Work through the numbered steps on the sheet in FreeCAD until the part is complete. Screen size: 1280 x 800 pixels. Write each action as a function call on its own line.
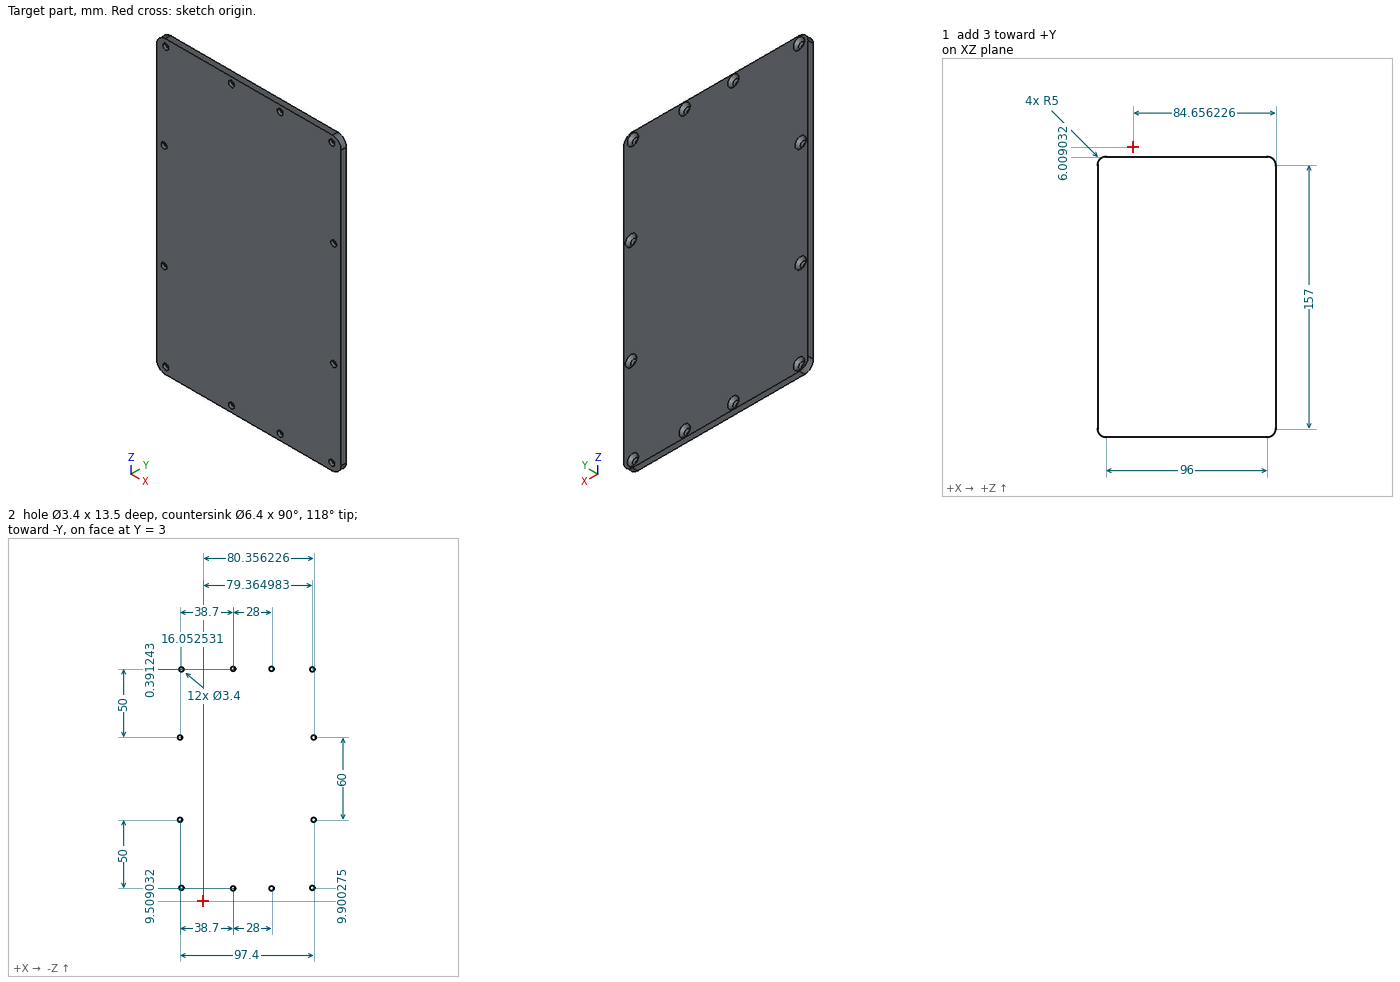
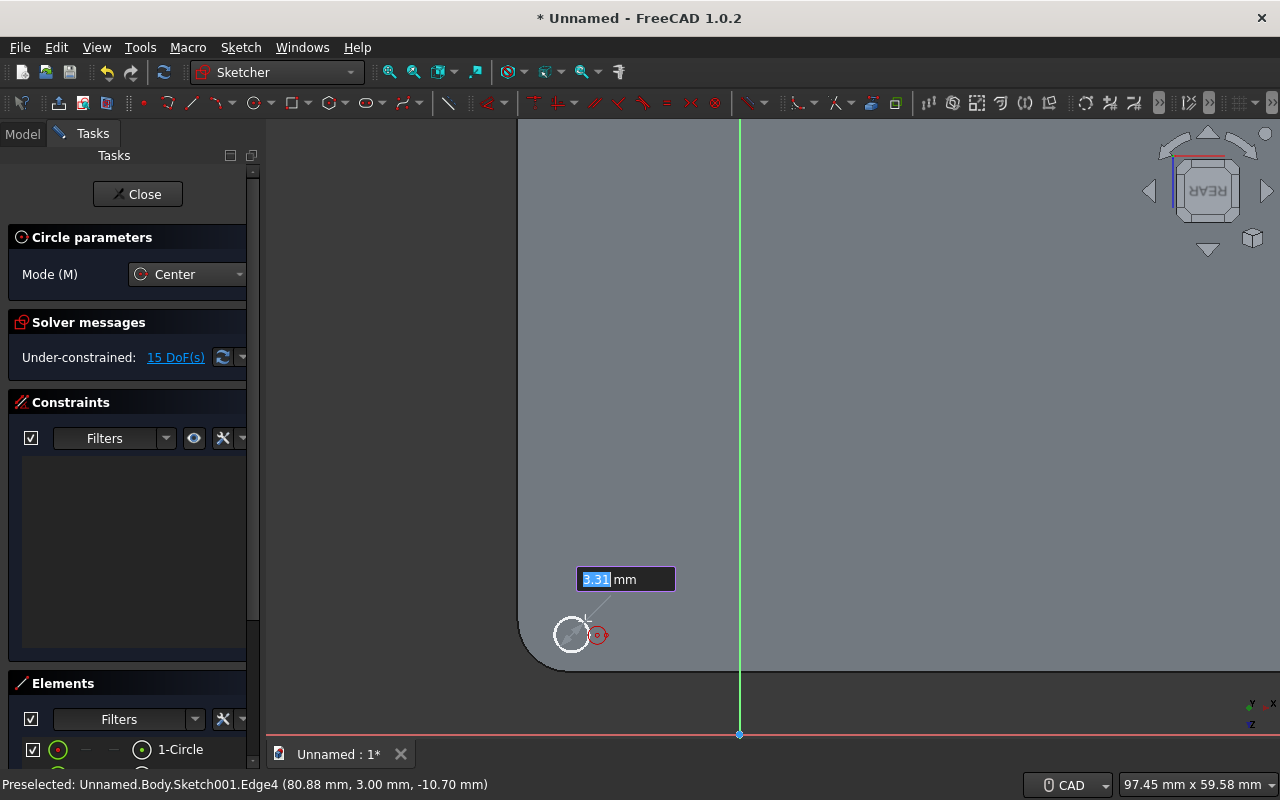
click(585, 619)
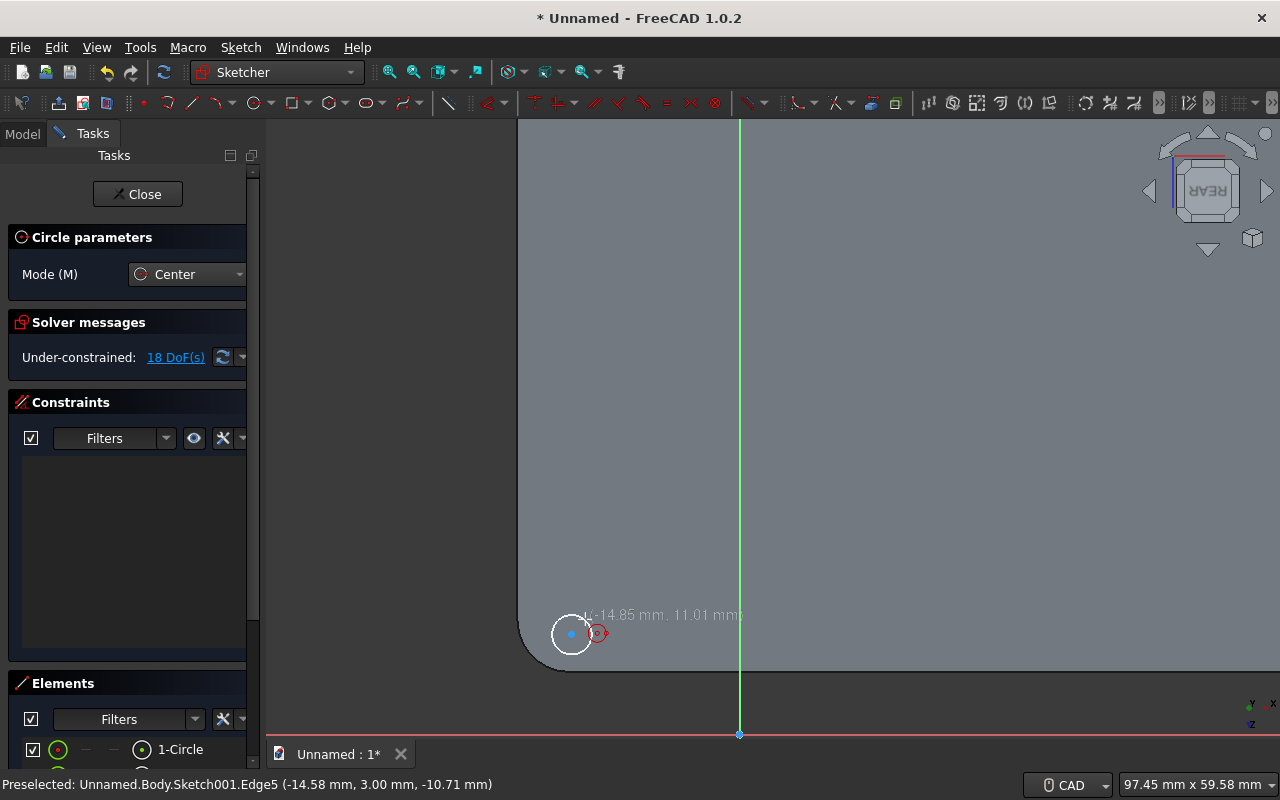
scroll(585, 621, down, 7)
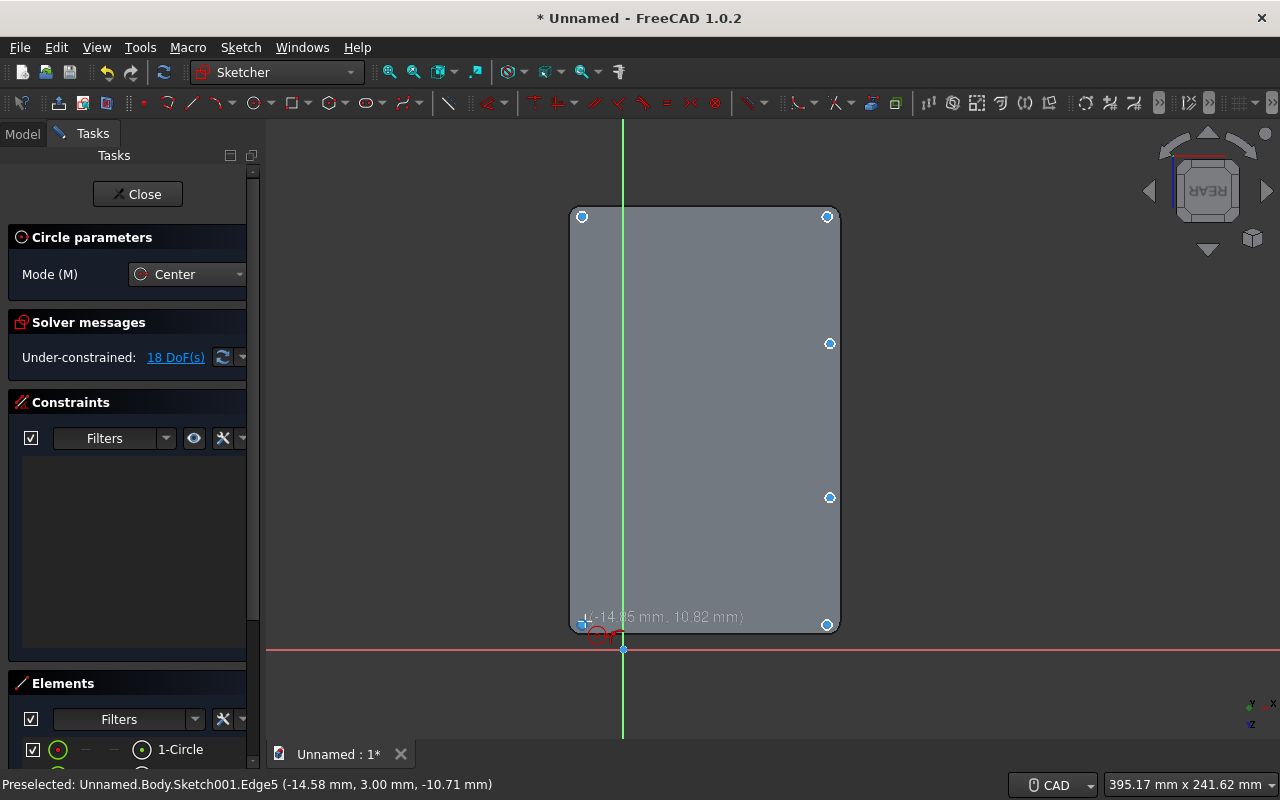
scroll(580, 497, up, 9)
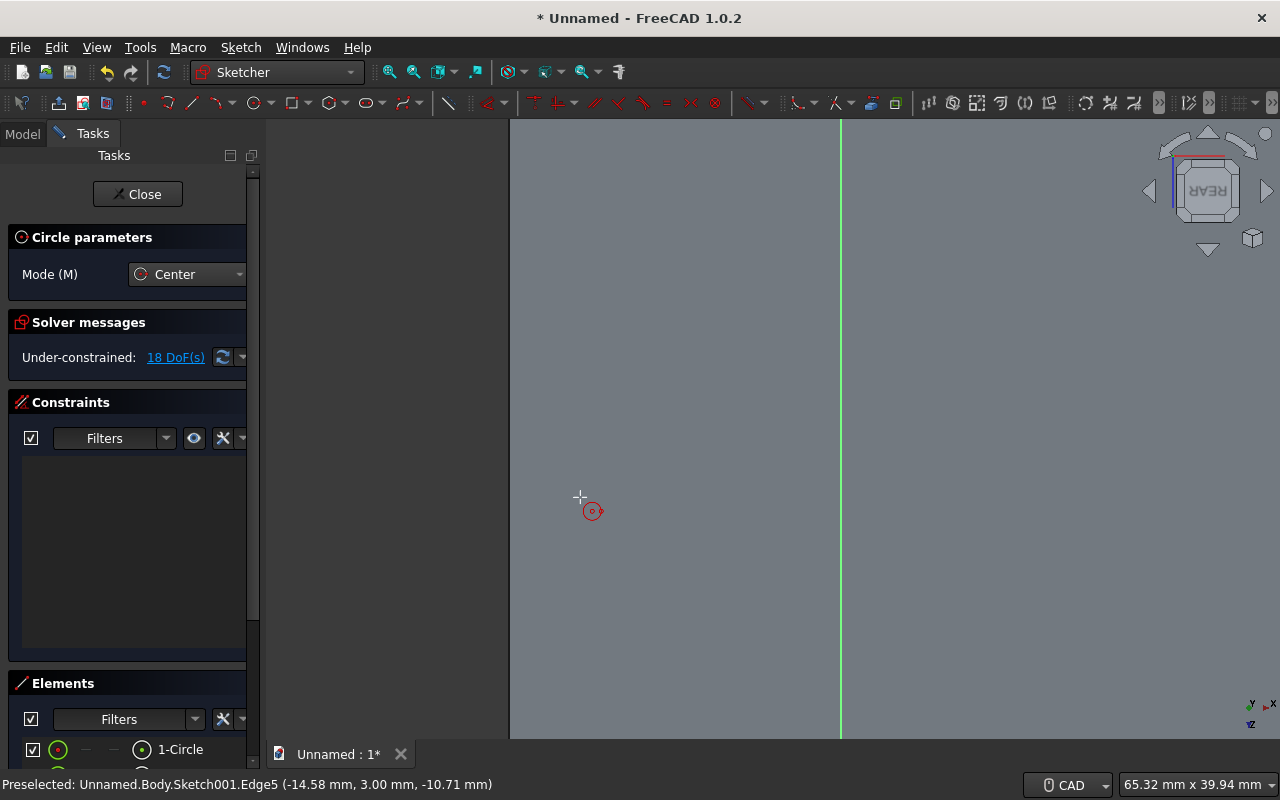
scroll(580, 496, down, 9)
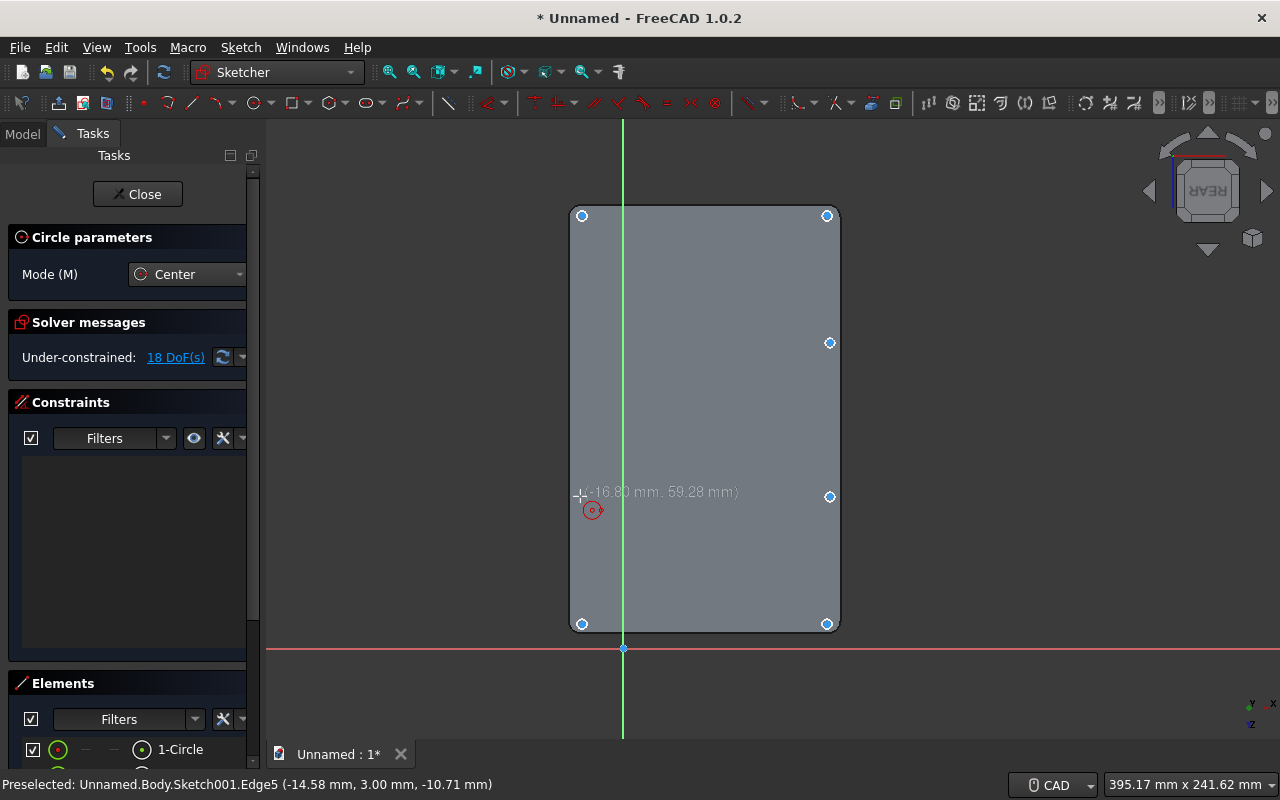
click(580, 496)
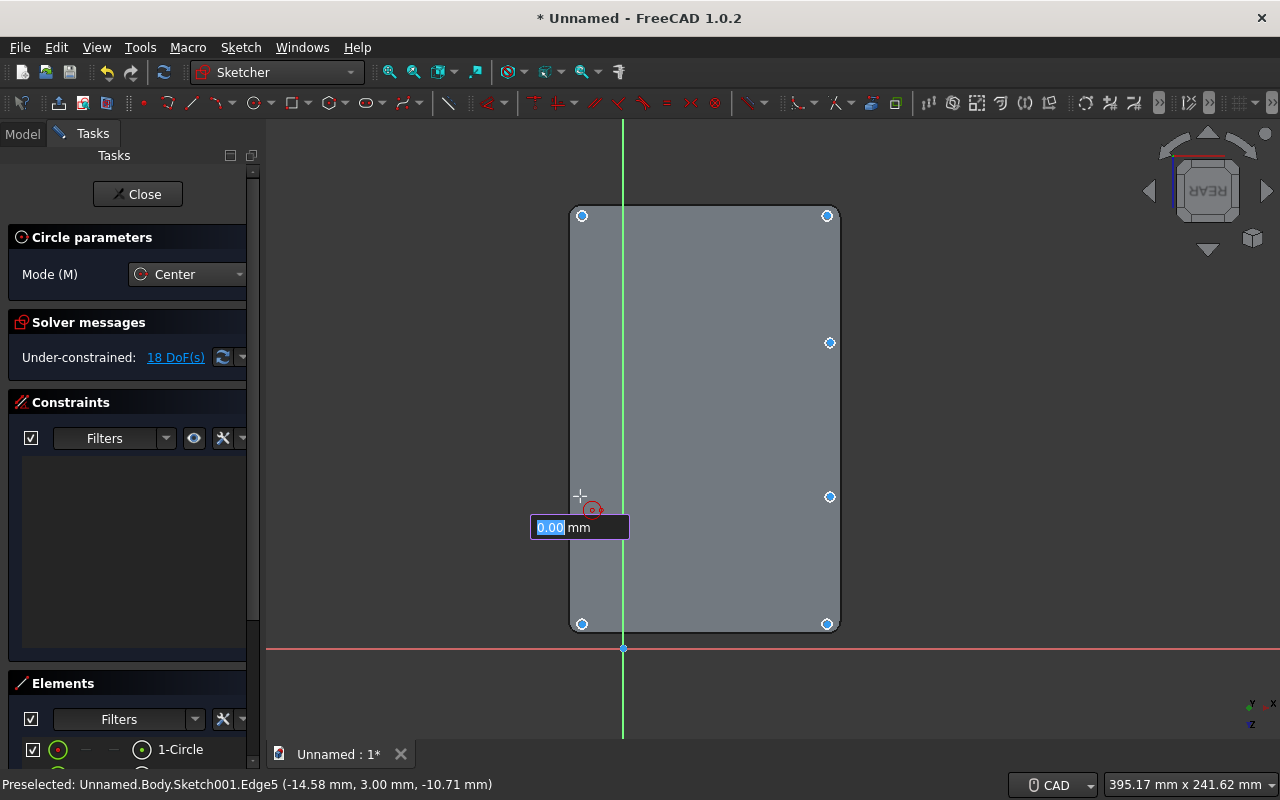
scroll(583, 493, up, 7)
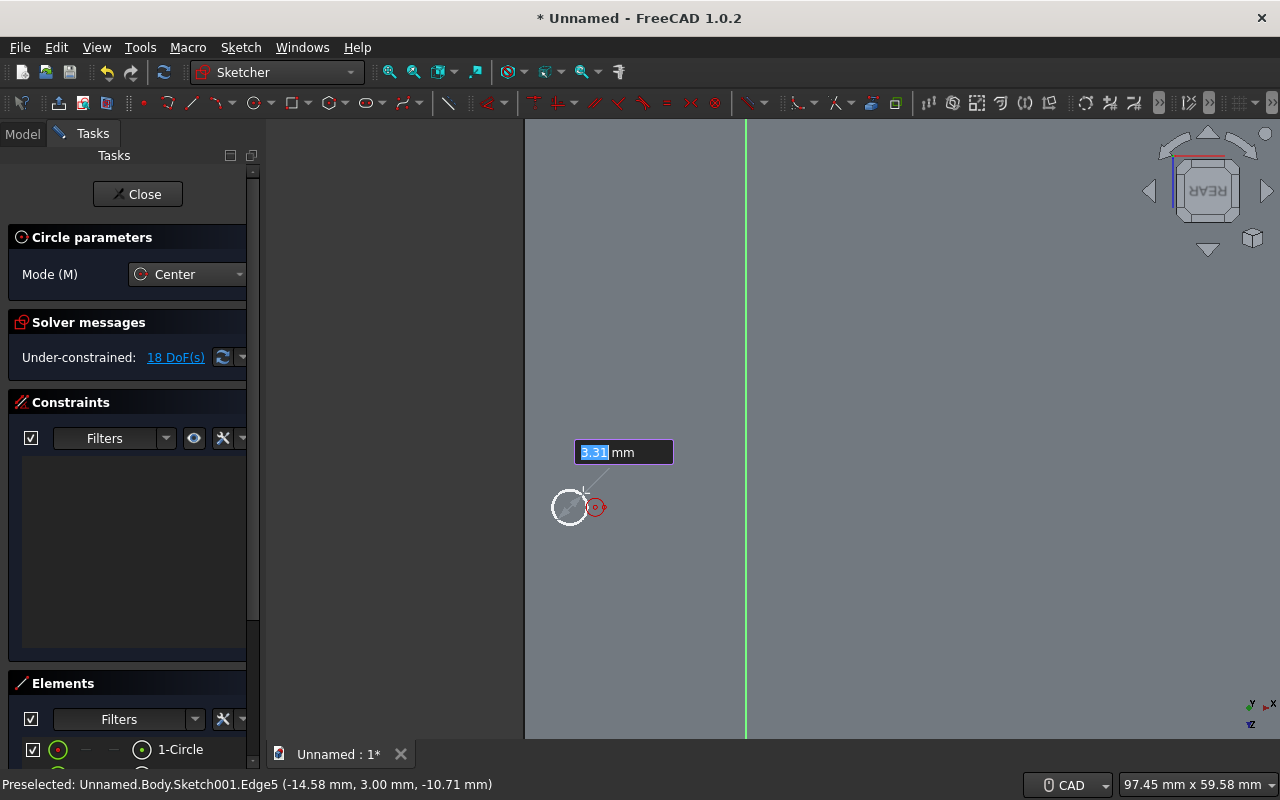
click(581, 491)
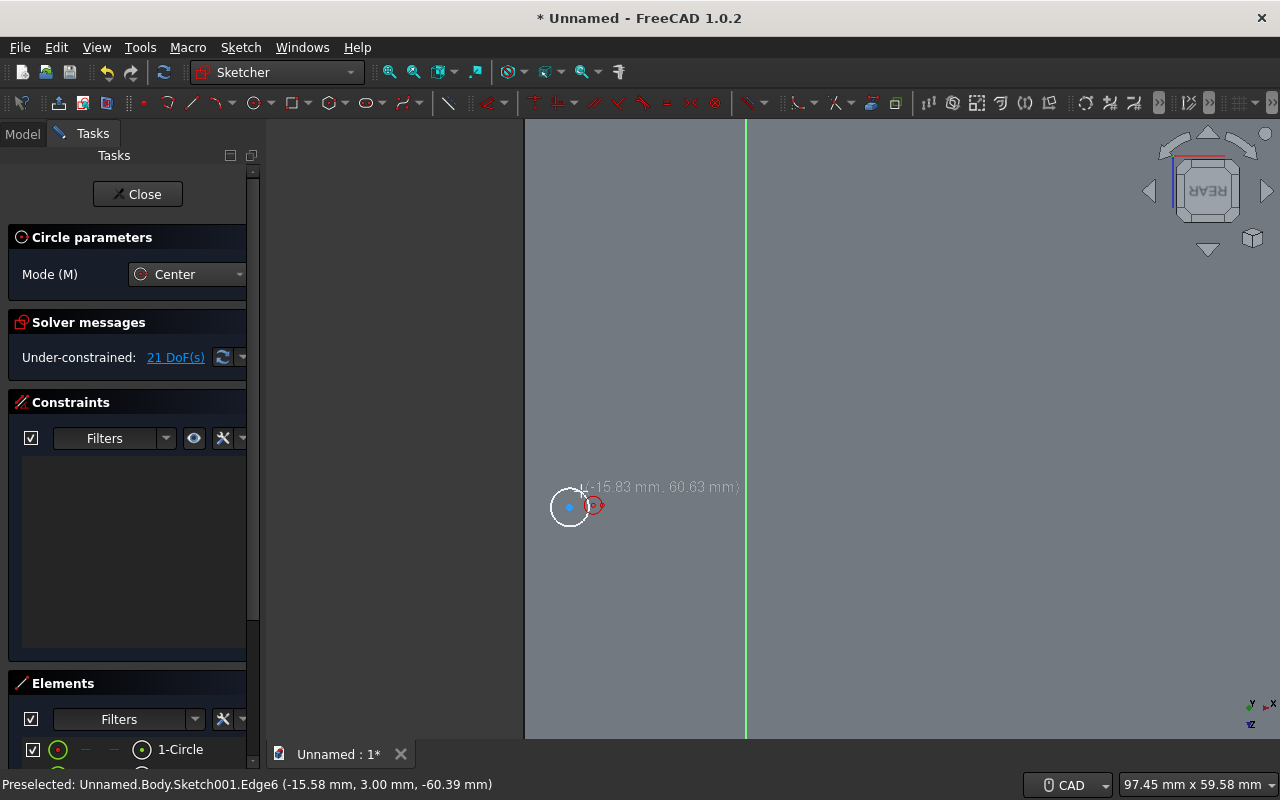
scroll(583, 493, down, 7)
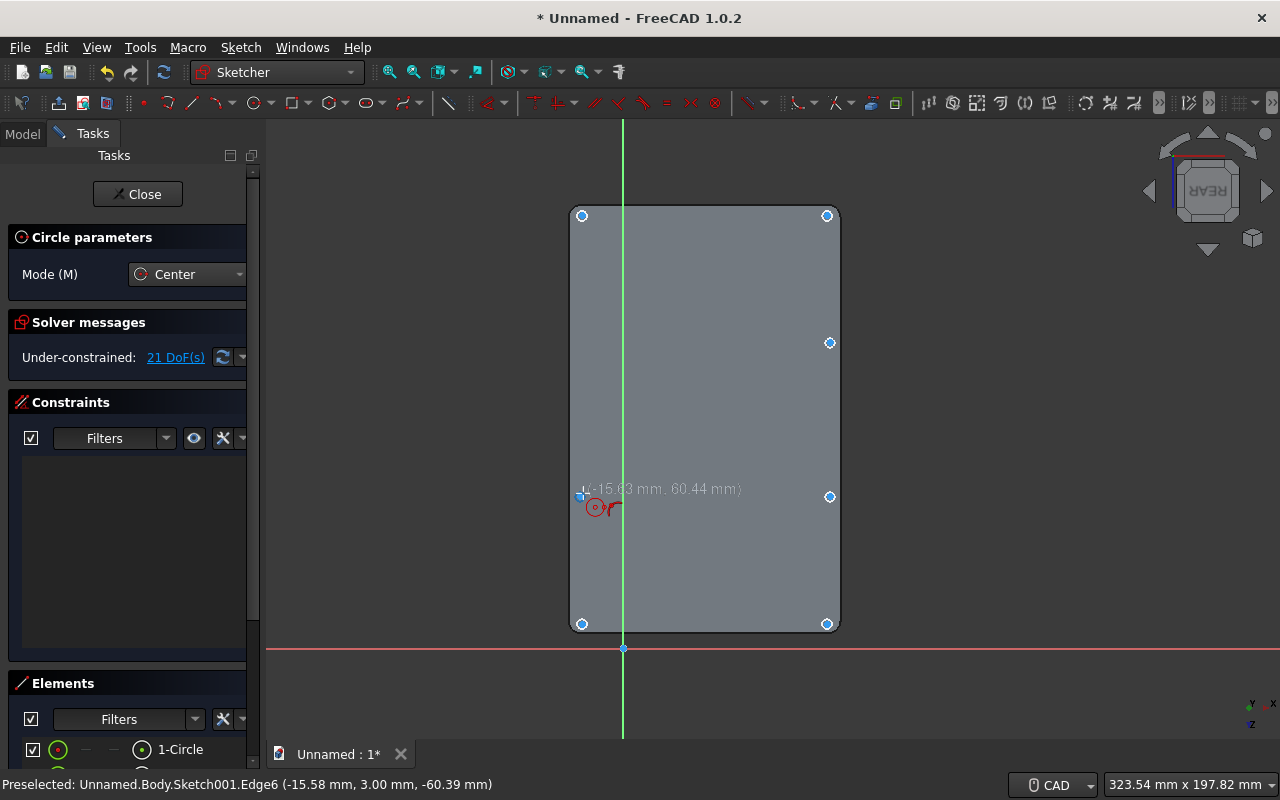
scroll(580, 342, up, 9)